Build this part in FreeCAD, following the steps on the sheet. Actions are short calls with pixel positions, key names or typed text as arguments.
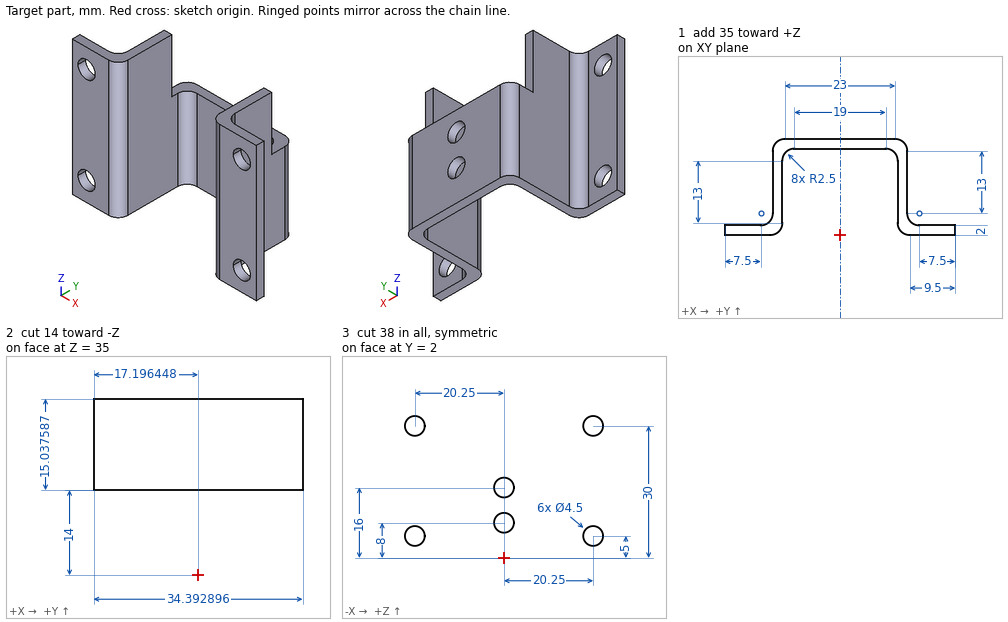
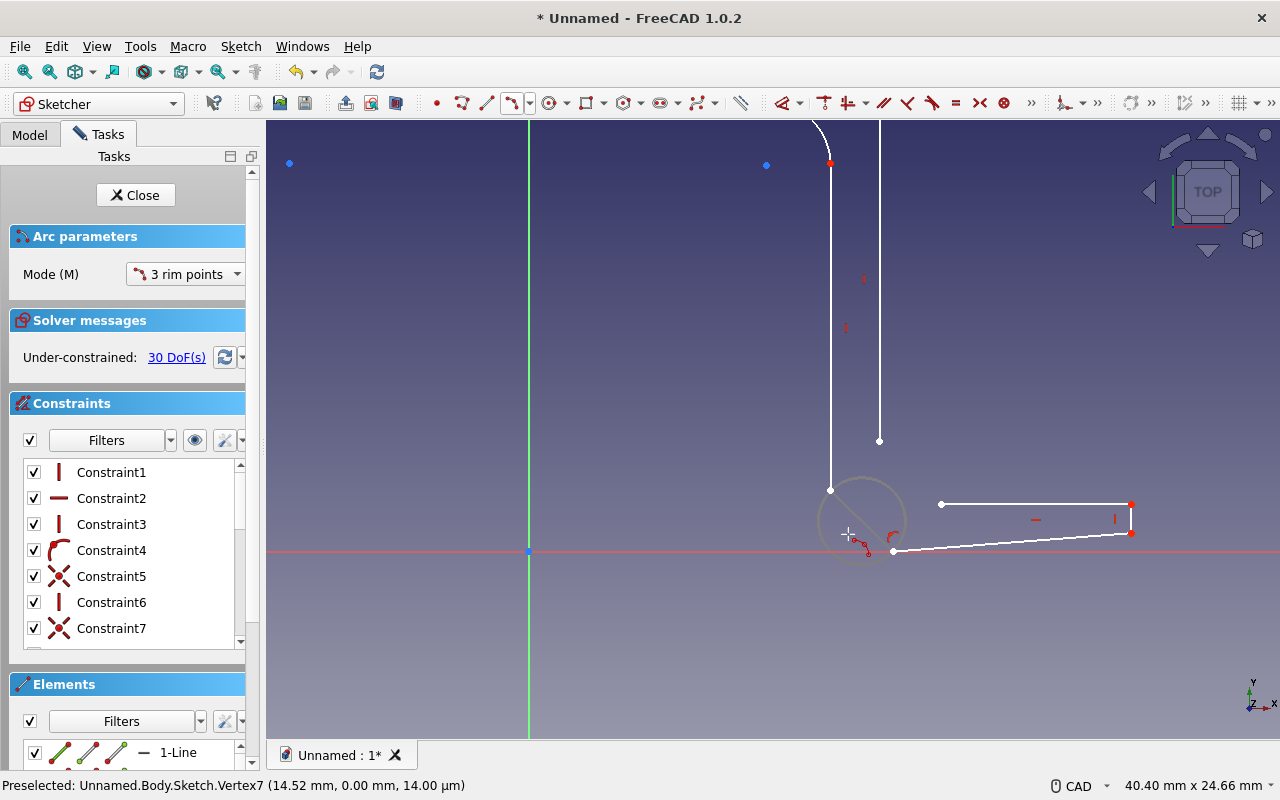
click(848, 533)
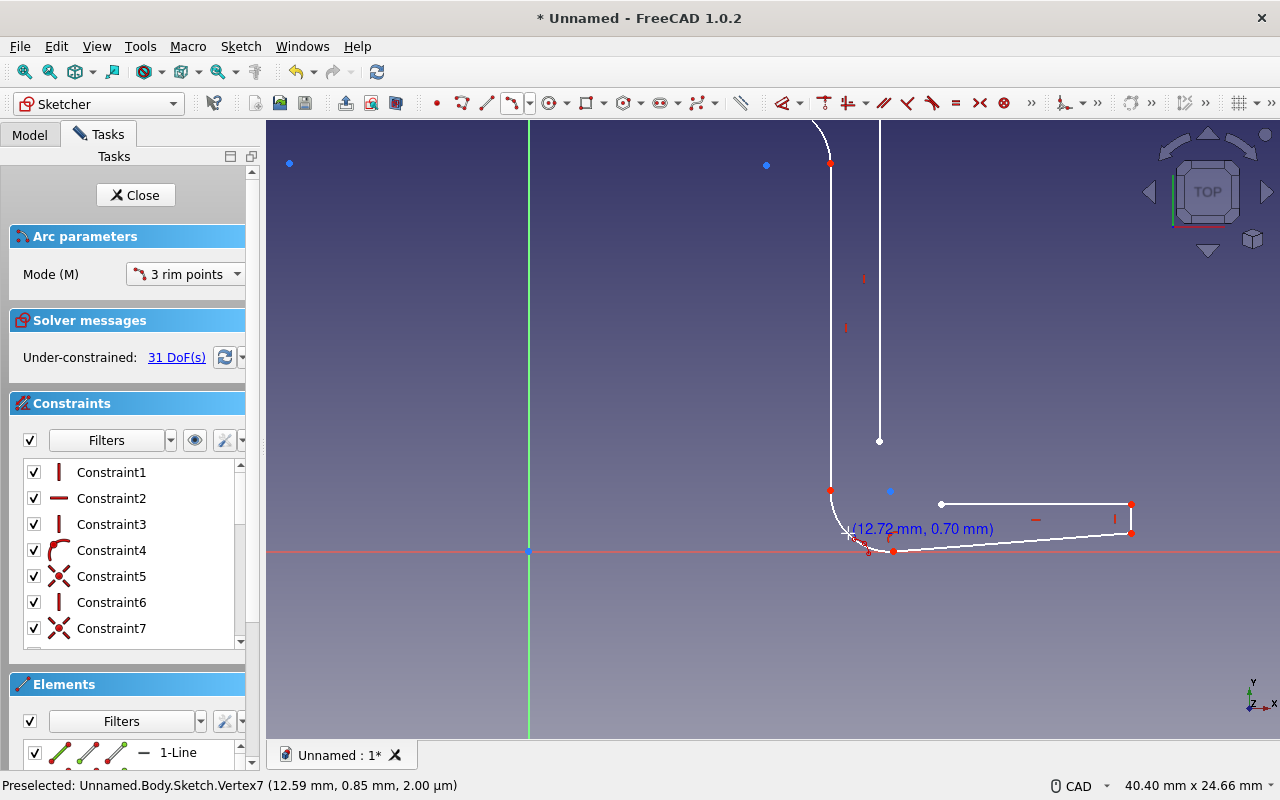
click(942, 504)
click(880, 442)
click(887, 467)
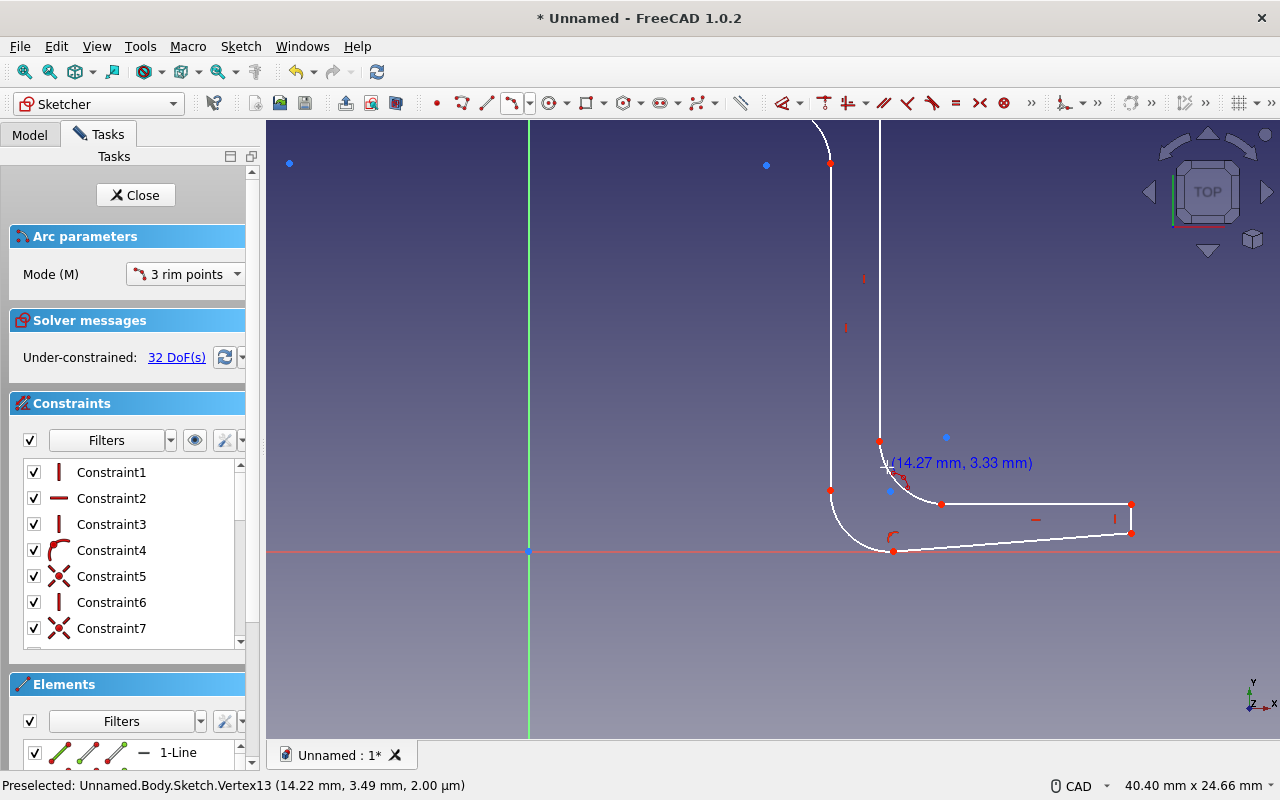
scroll(848, 535, down, 4)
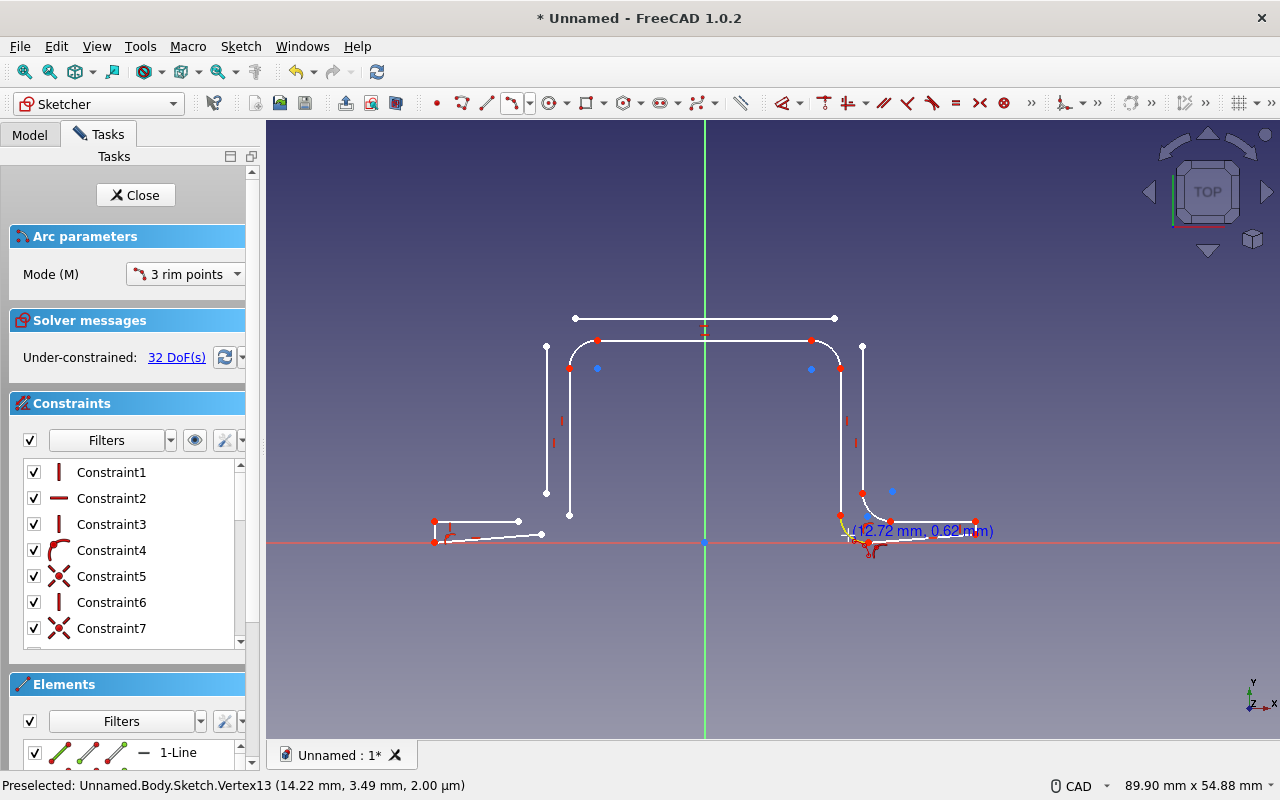
click(863, 347)
click(835, 319)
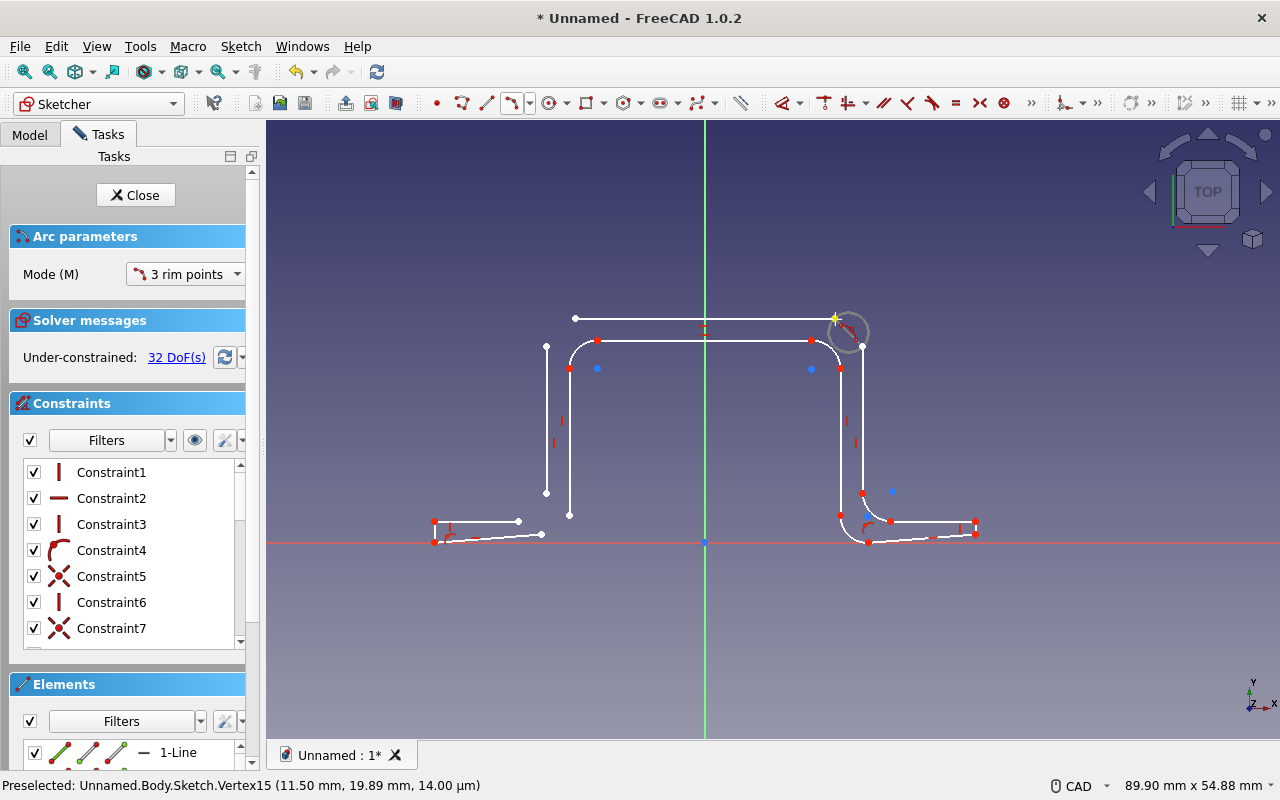
scroll(854, 326, up, 4)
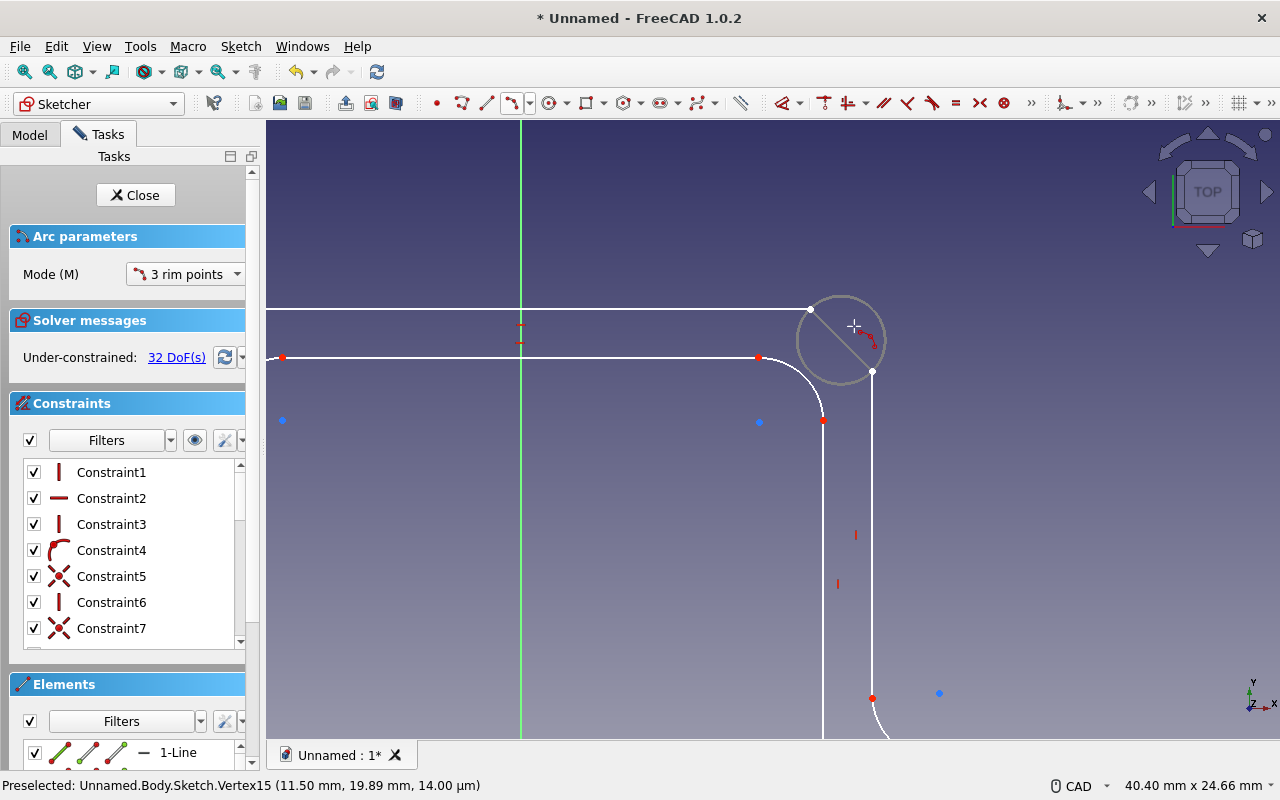
click(854, 325)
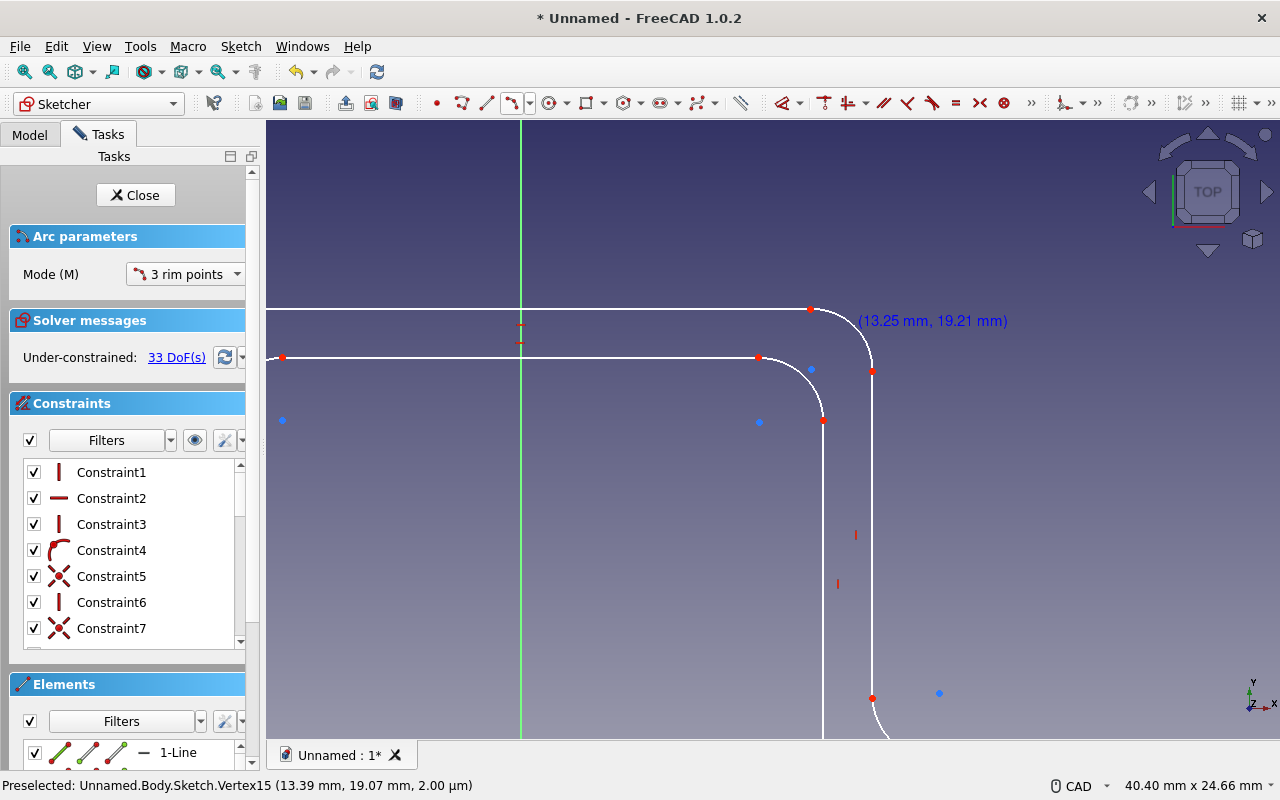
scroll(854, 325, down, 4)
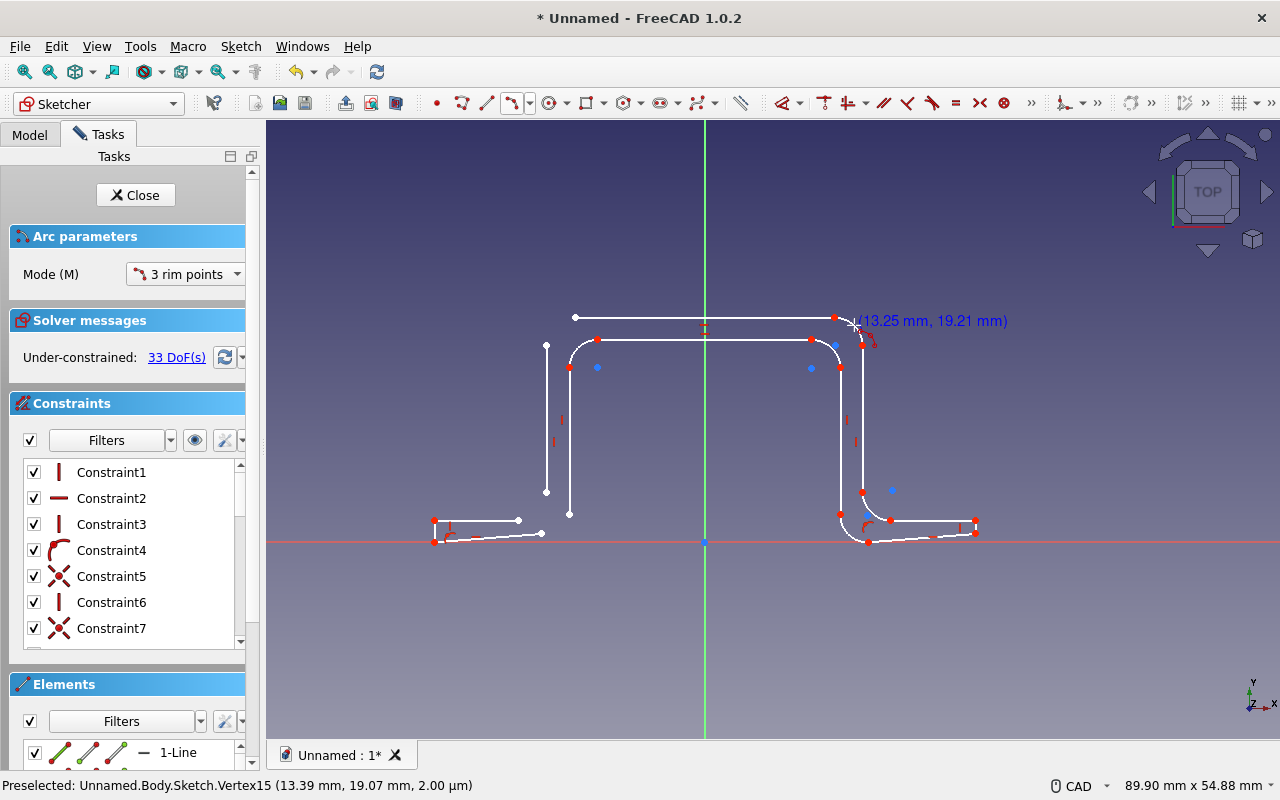
click(576, 318)
click(547, 346)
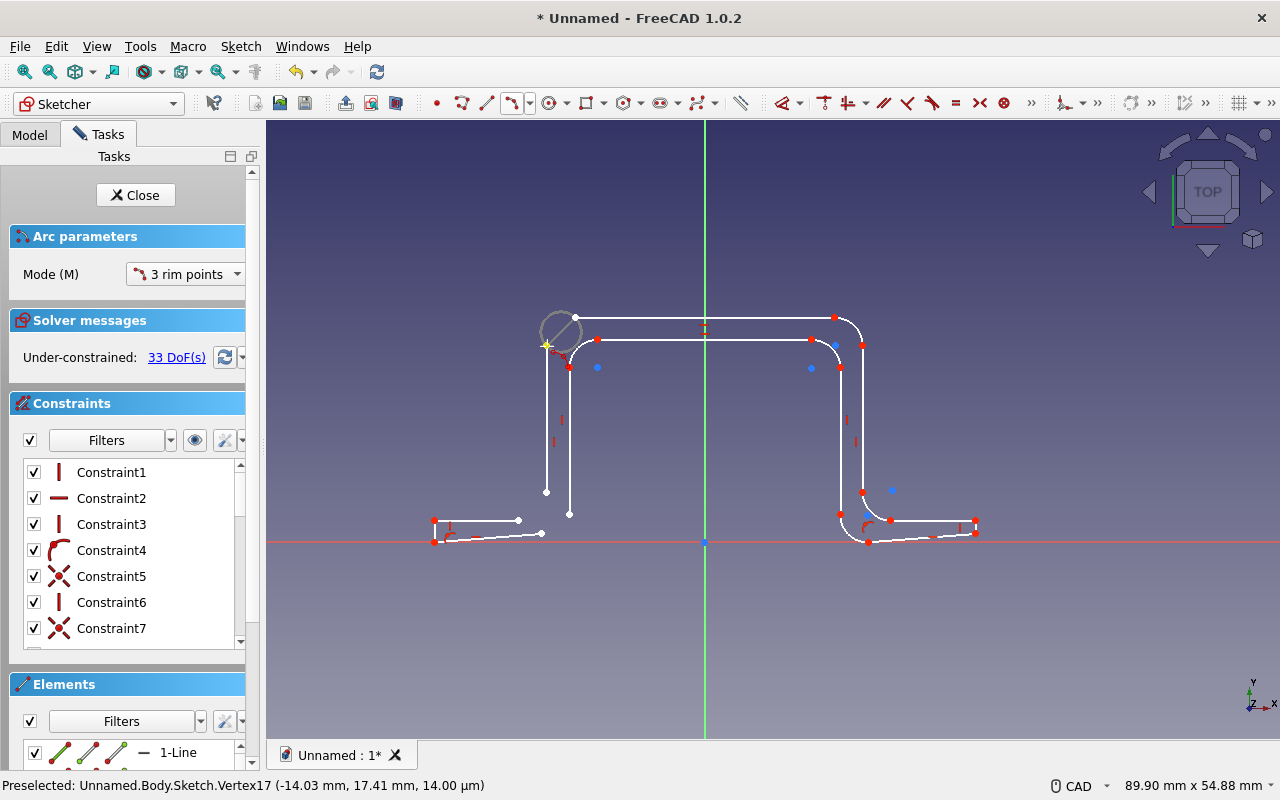
scroll(555, 325, up, 4)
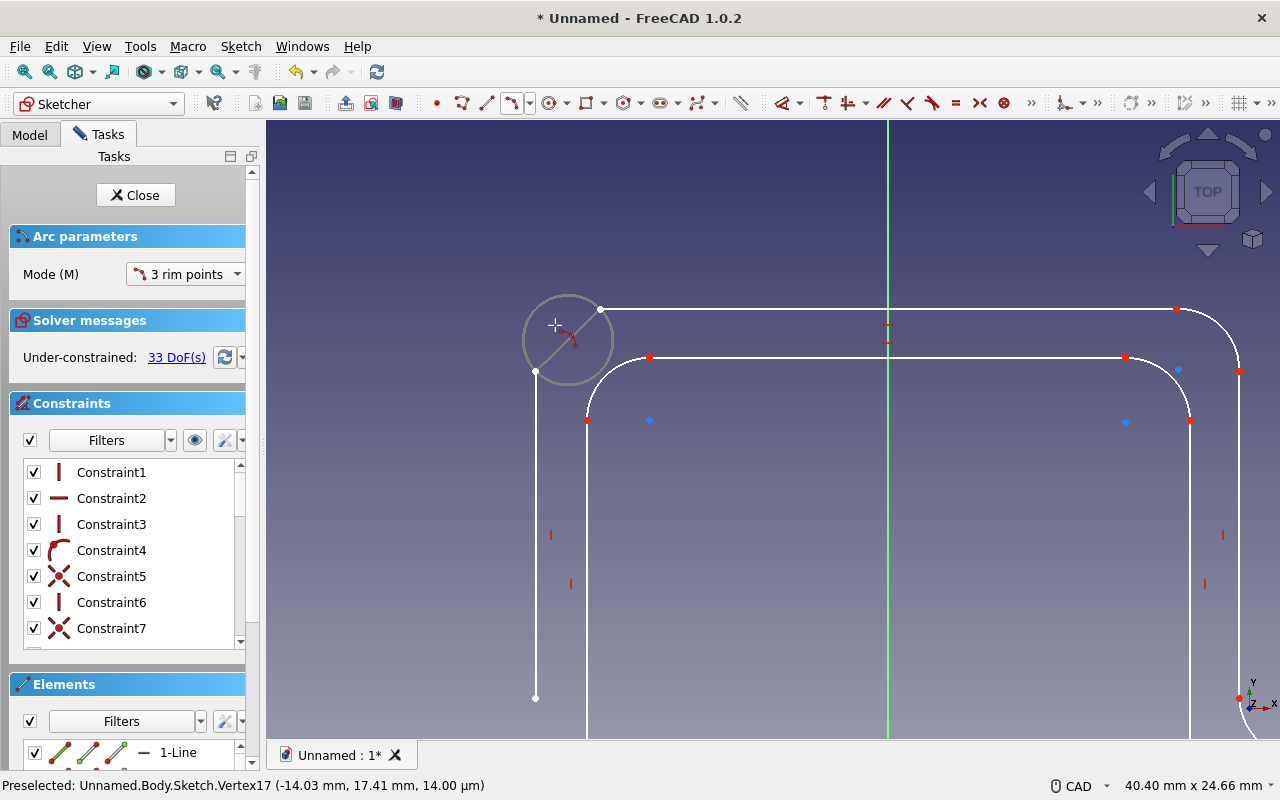
click(555, 325)